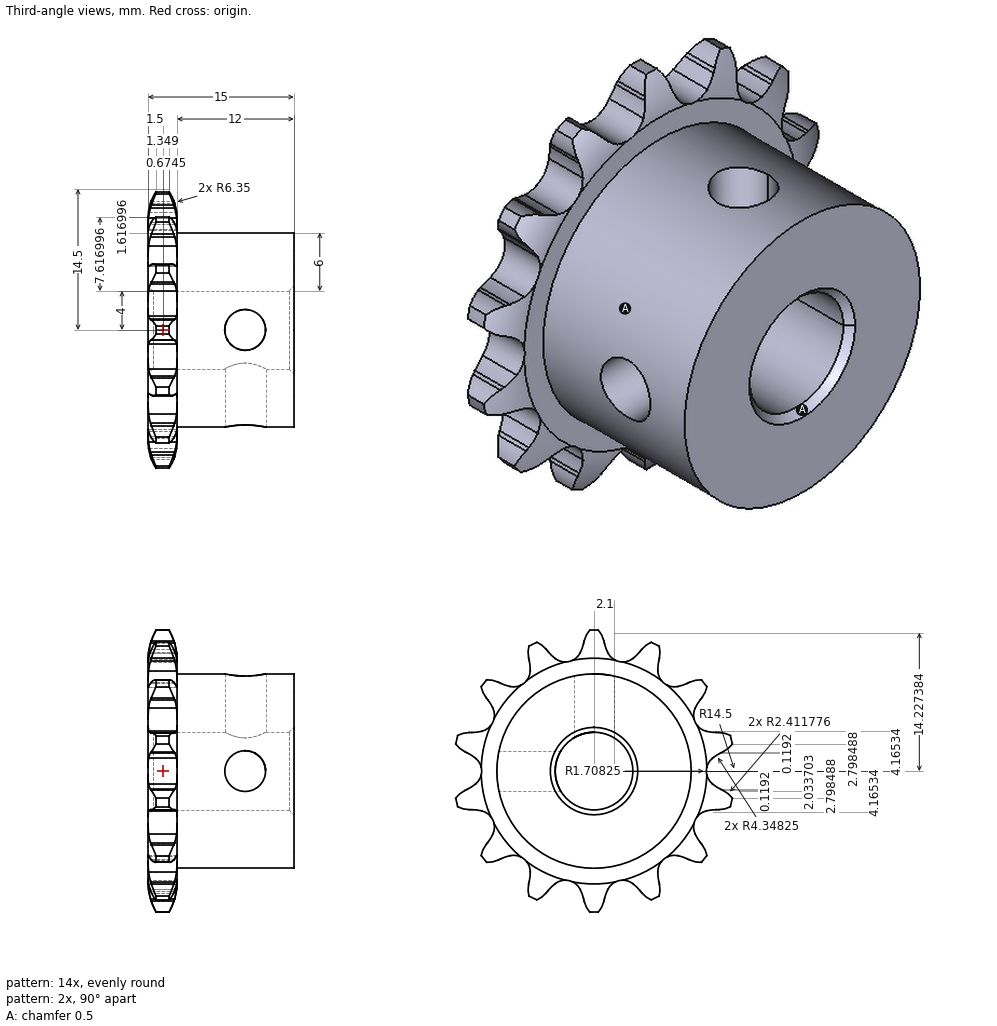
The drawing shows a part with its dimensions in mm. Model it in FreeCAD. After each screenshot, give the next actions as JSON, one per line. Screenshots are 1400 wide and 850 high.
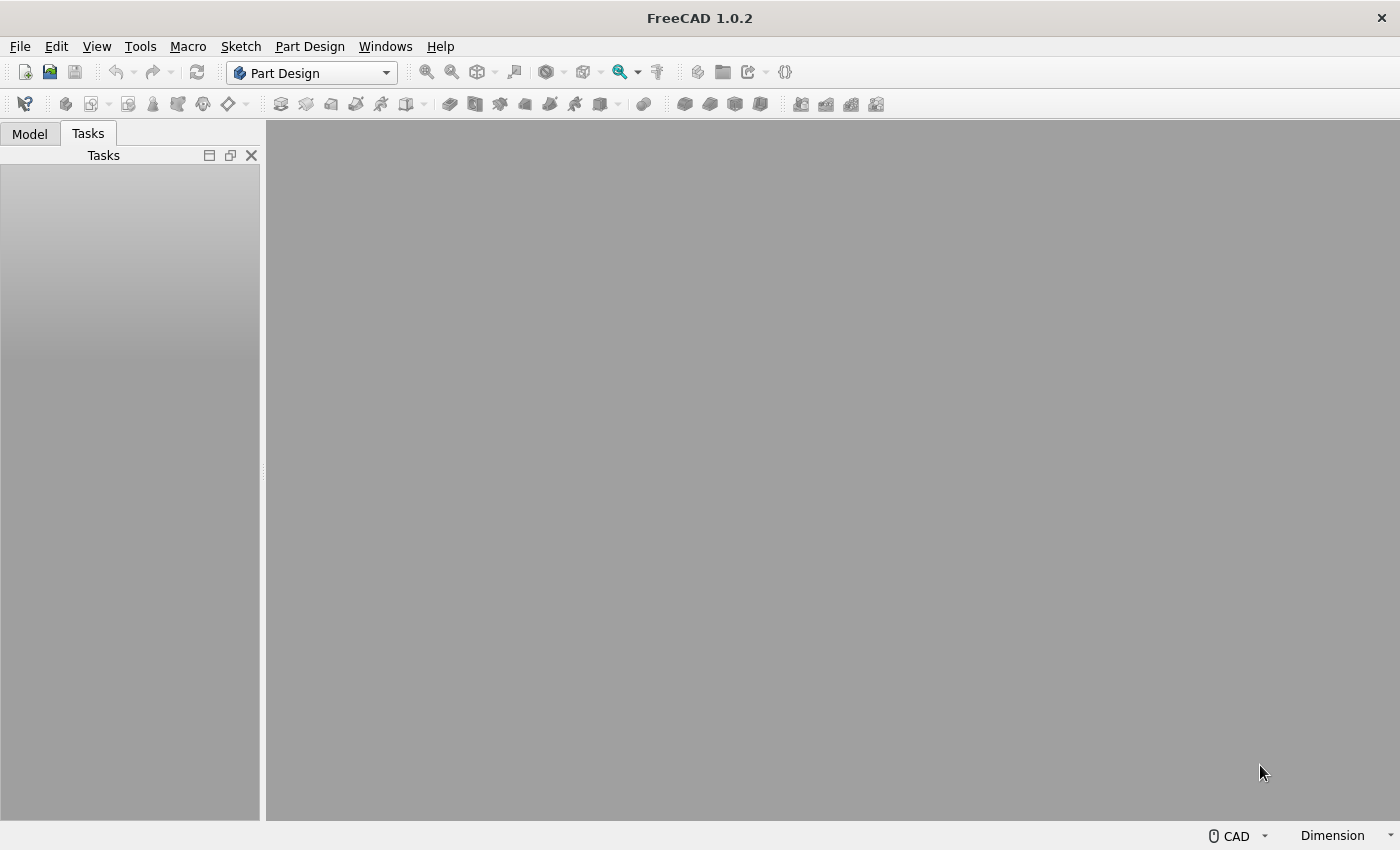
{"action": "left_click", "coordinate": [25, 72]}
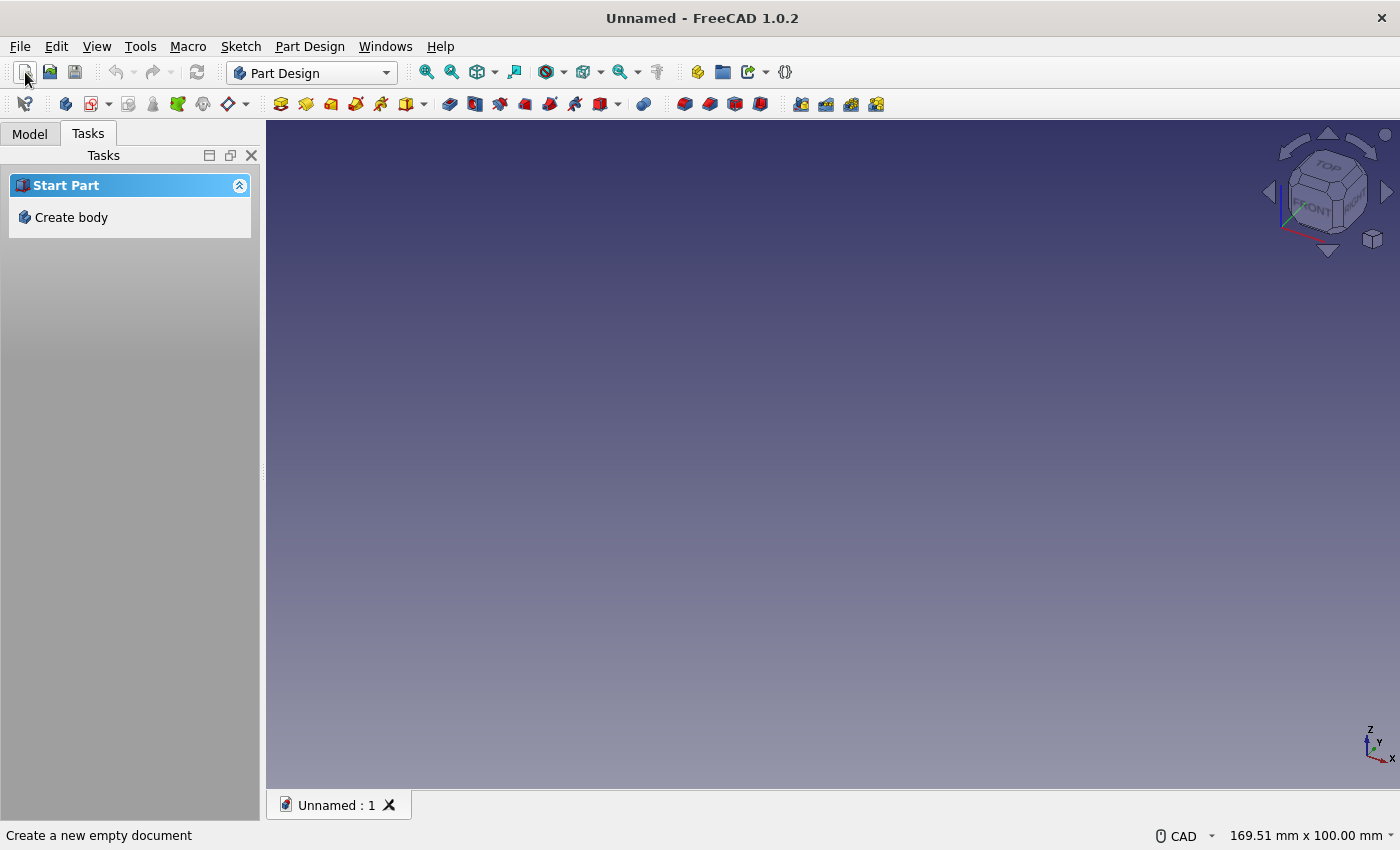
{"action": "left_click", "coordinate": [90, 104]}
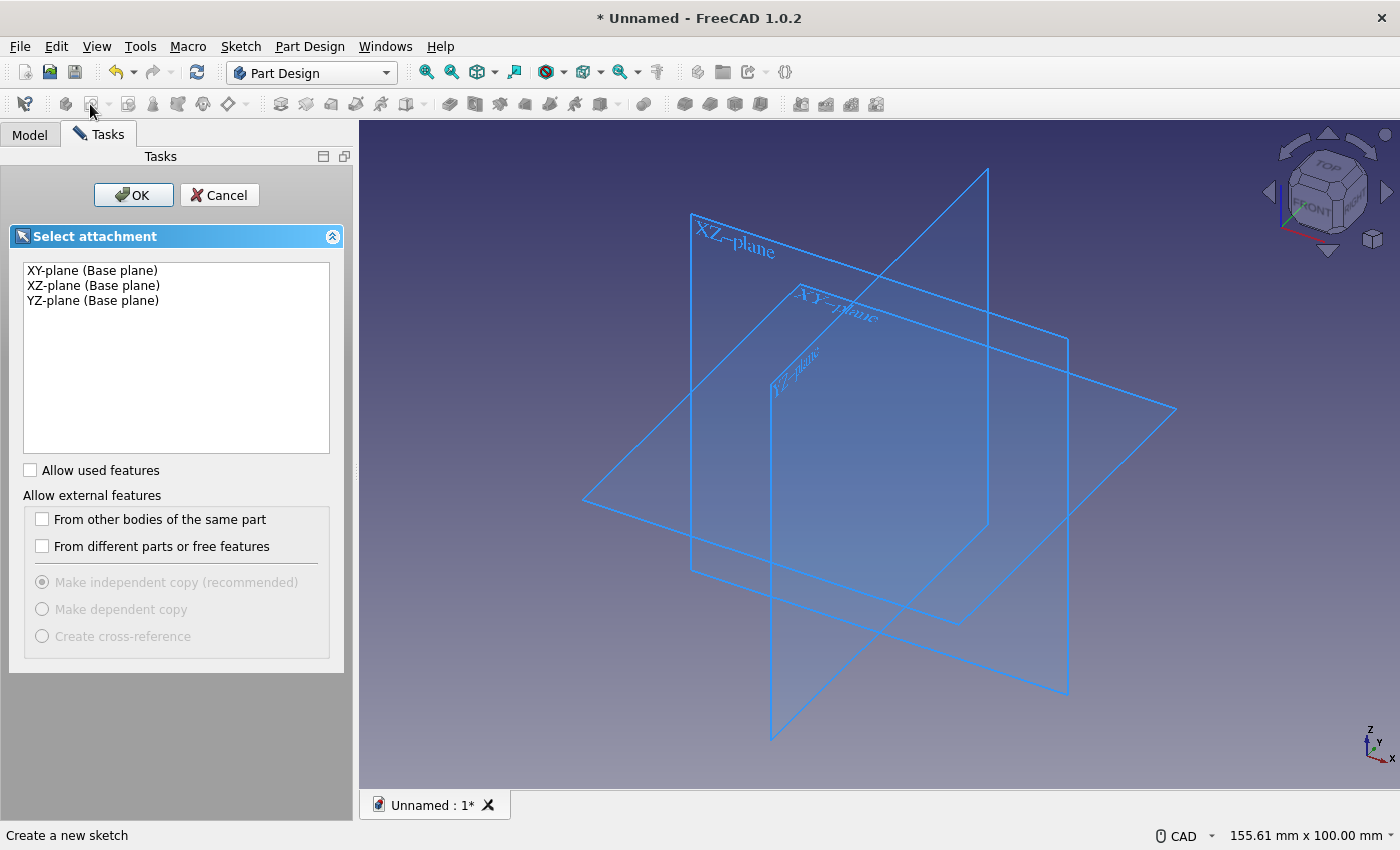
{"action": "left_click", "coordinate": [84, 270]}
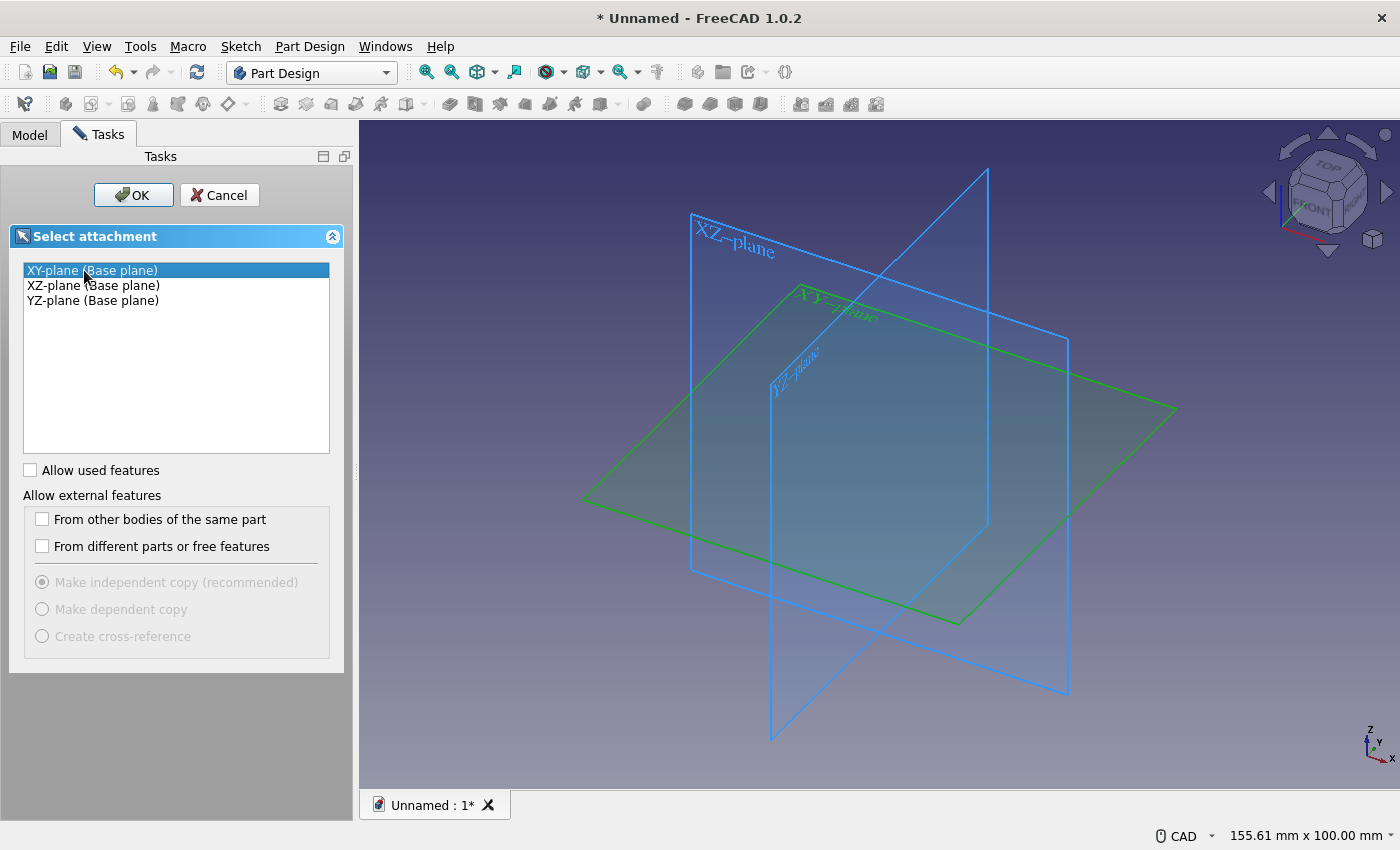
{"action": "left_click", "coordinate": [134, 195]}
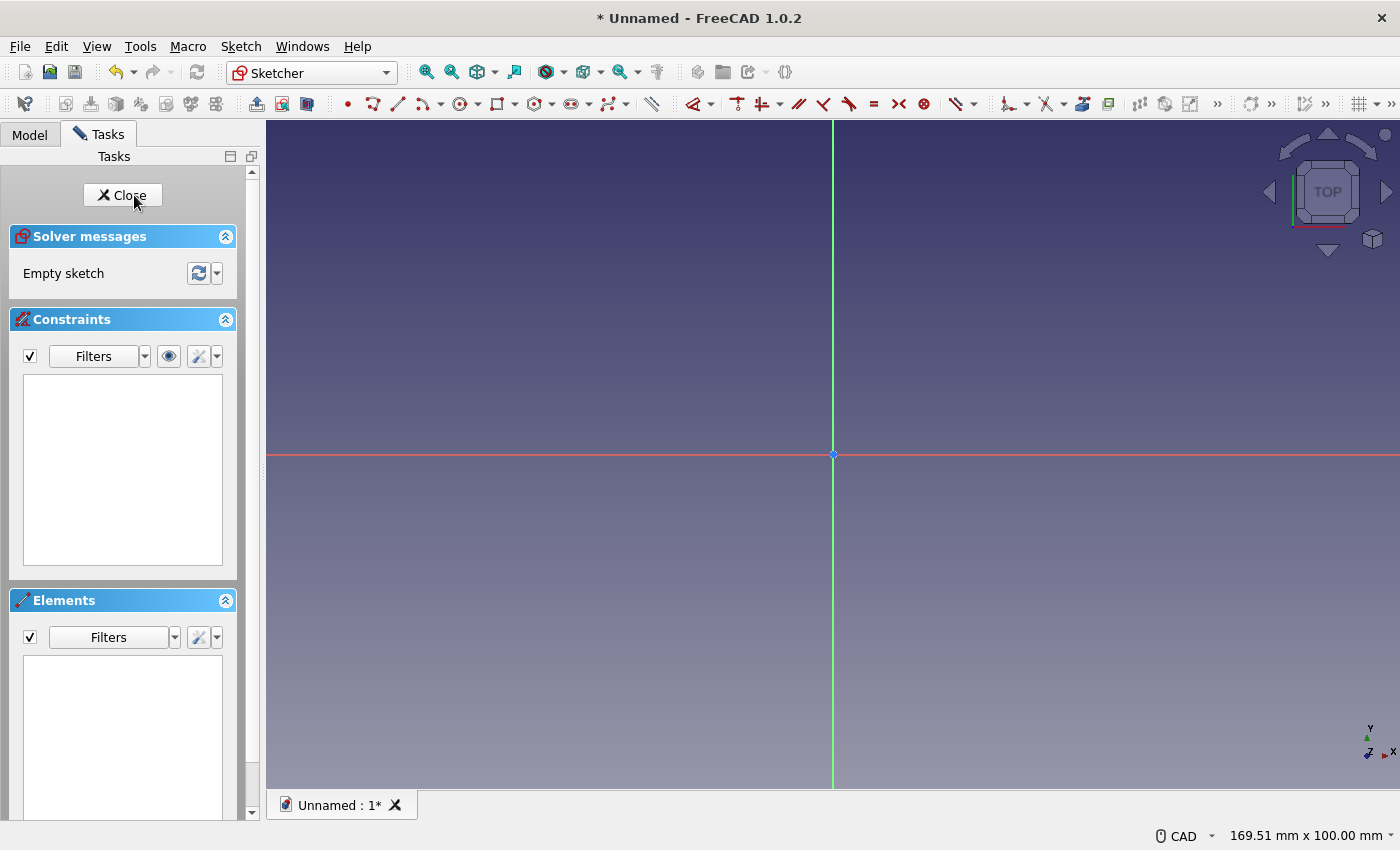
{"action": "scroll", "coordinate": [909, 390], "scroll_direction": "up", "scroll_amount": 7}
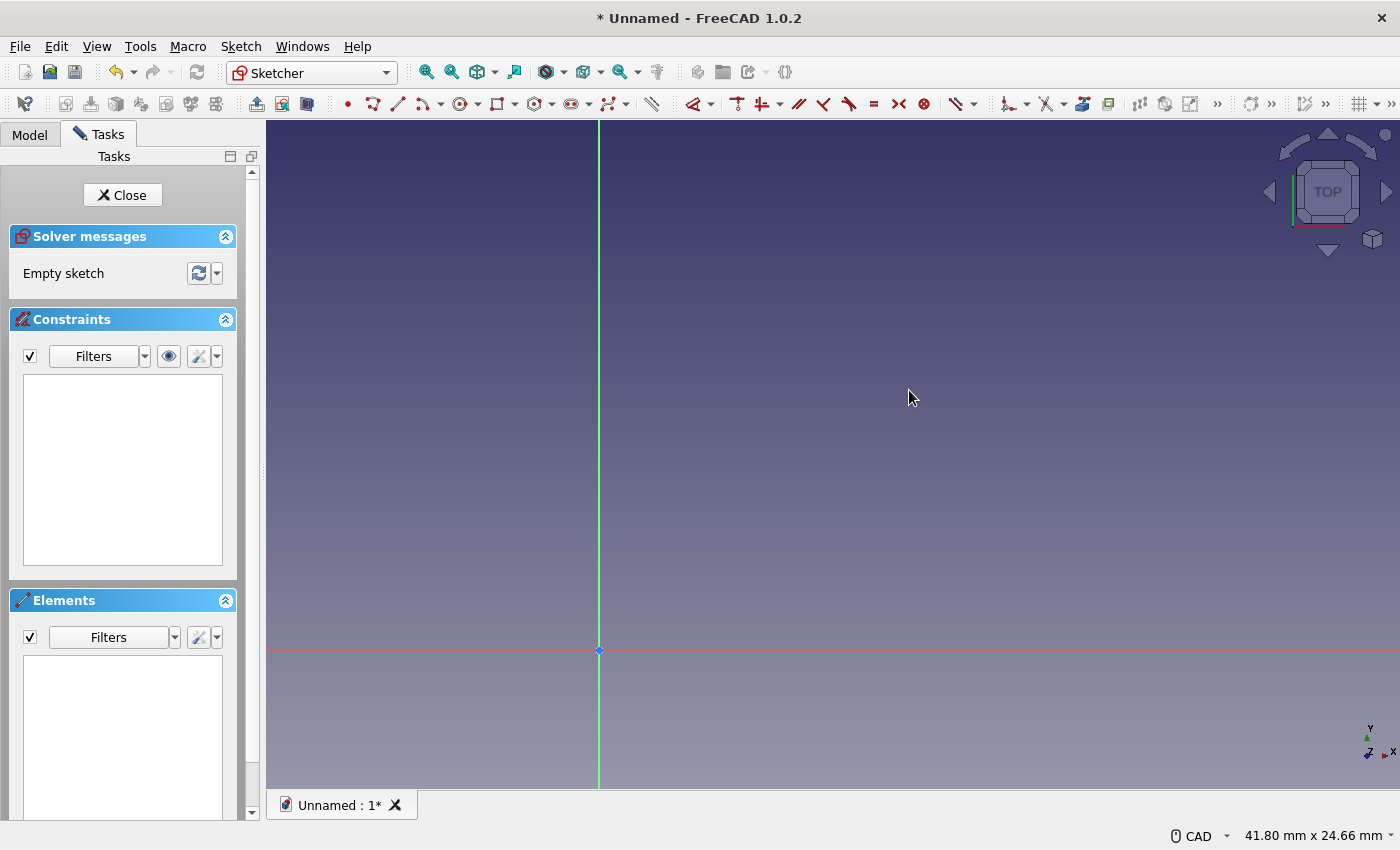
{"action": "left_click", "coordinate": [373, 104]}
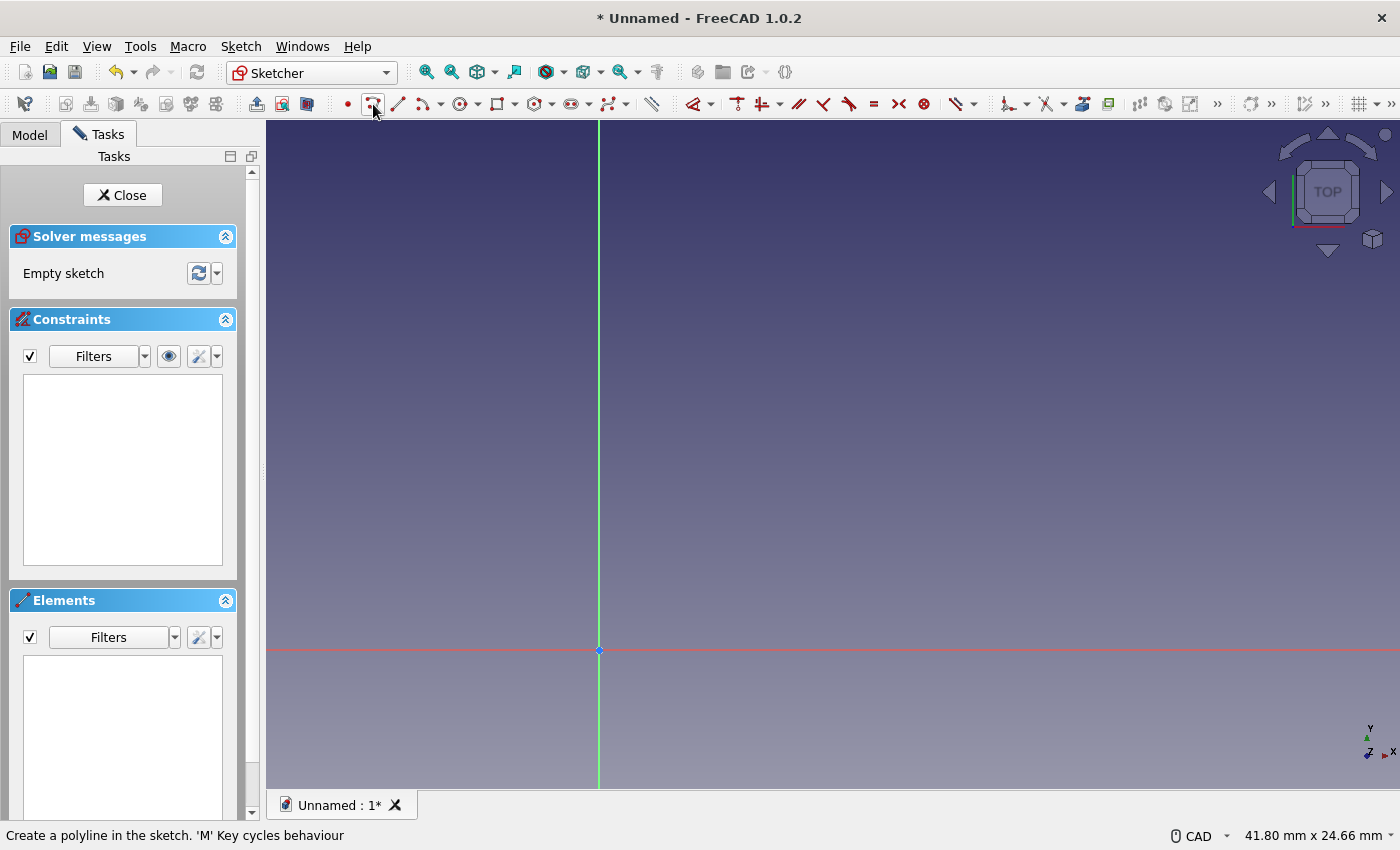
{"action": "left_click", "coordinate": [558, 335]}
{"action": "left_click", "coordinate": [558, 542]}
{"action": "left_click", "coordinate": [965, 542]}
{"action": "left_click", "coordinate": [965, 379]}
{"action": "left_click", "coordinate": [640, 379]}
{"action": "left_click", "coordinate": [640, 335]}
{"action": "right_click", "coordinate": [640, 335]}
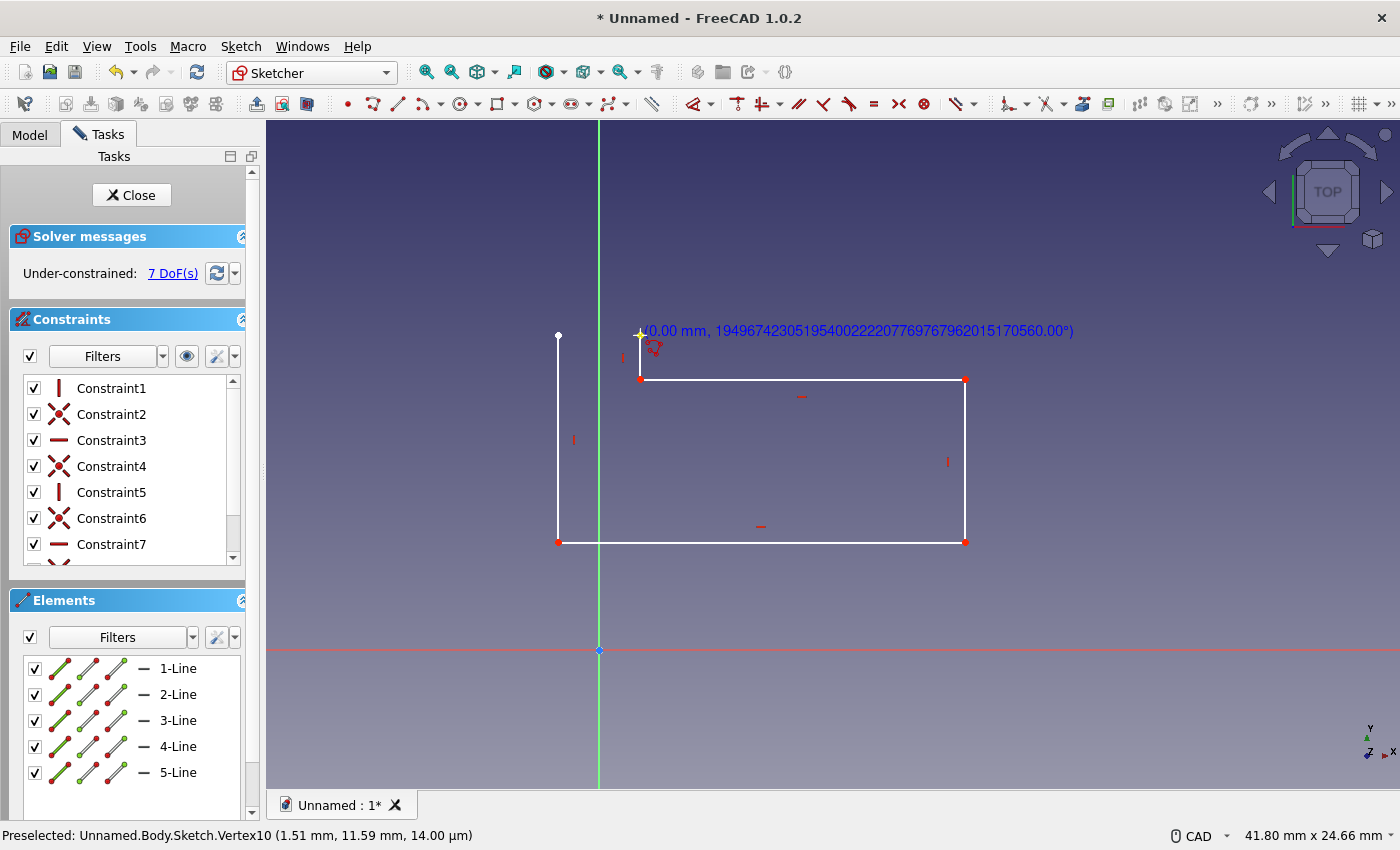
{"action": "left_click", "coordinate": [398, 104]}